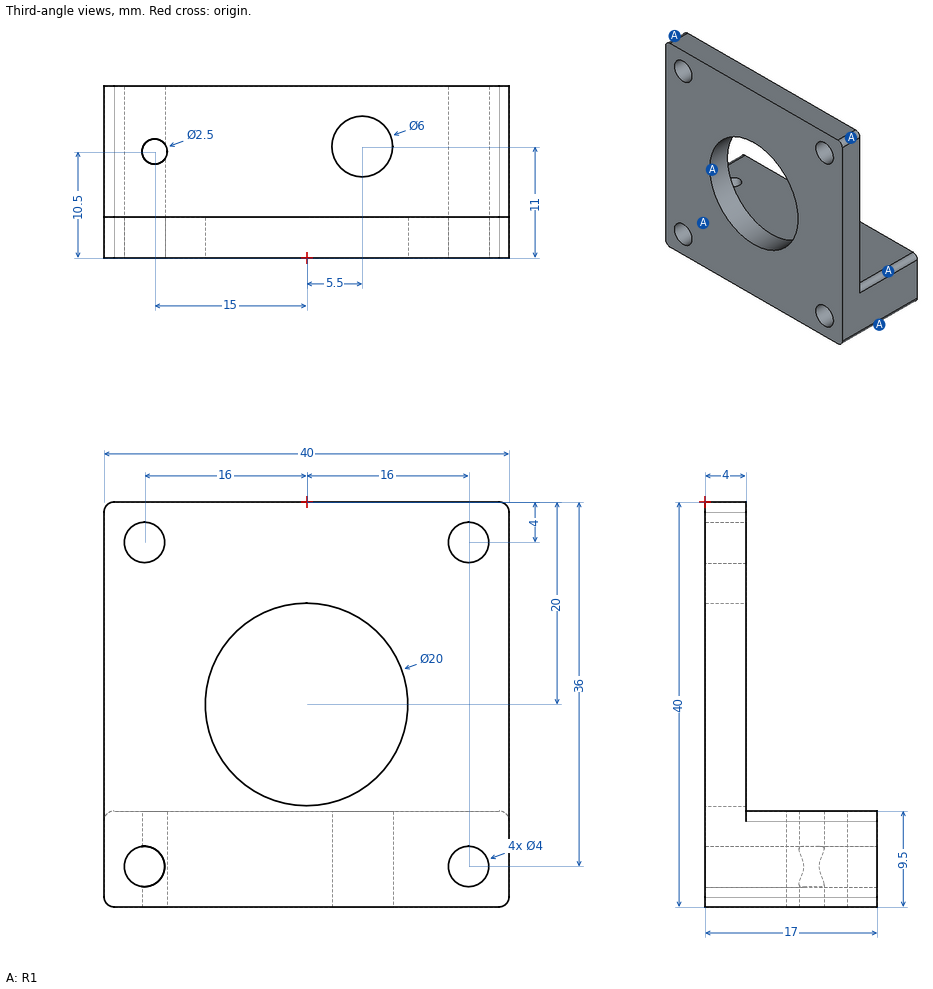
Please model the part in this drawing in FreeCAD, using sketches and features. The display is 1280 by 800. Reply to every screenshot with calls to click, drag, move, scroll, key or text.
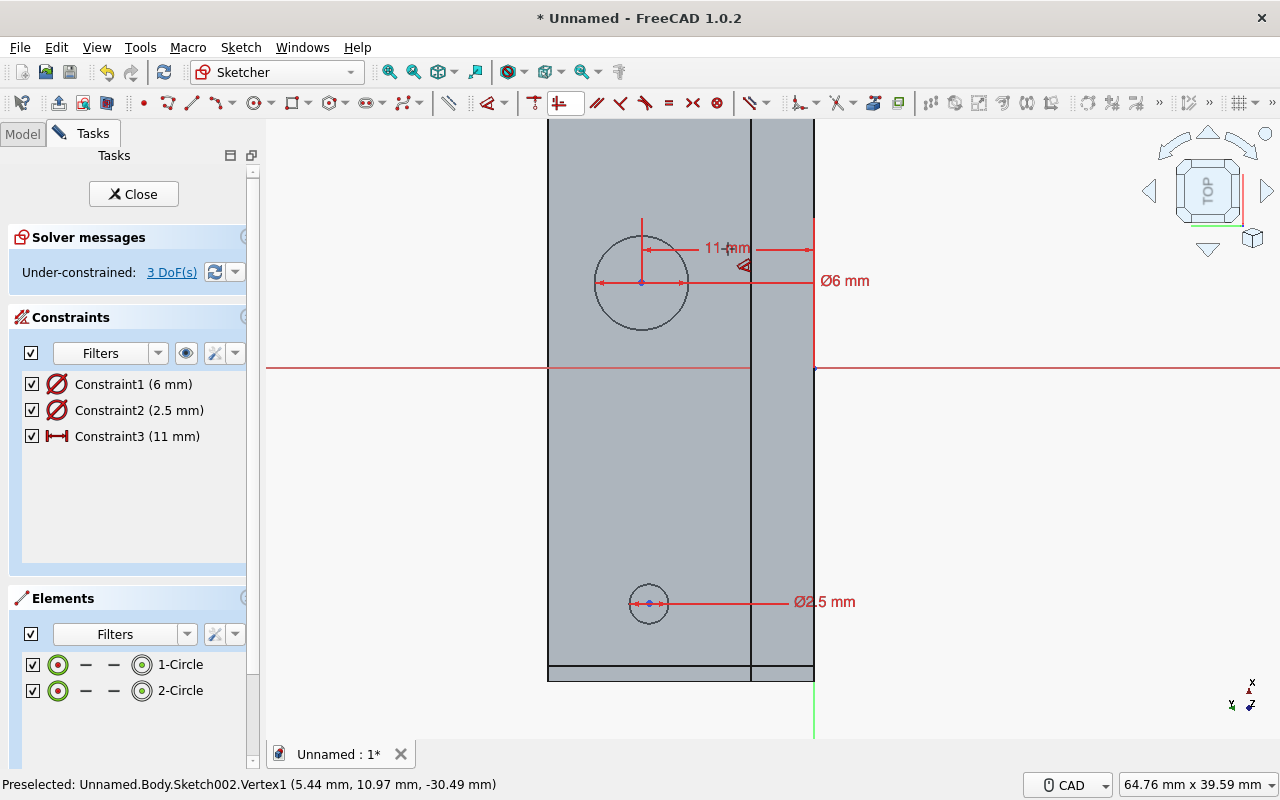
click(649, 604)
click(848, 486)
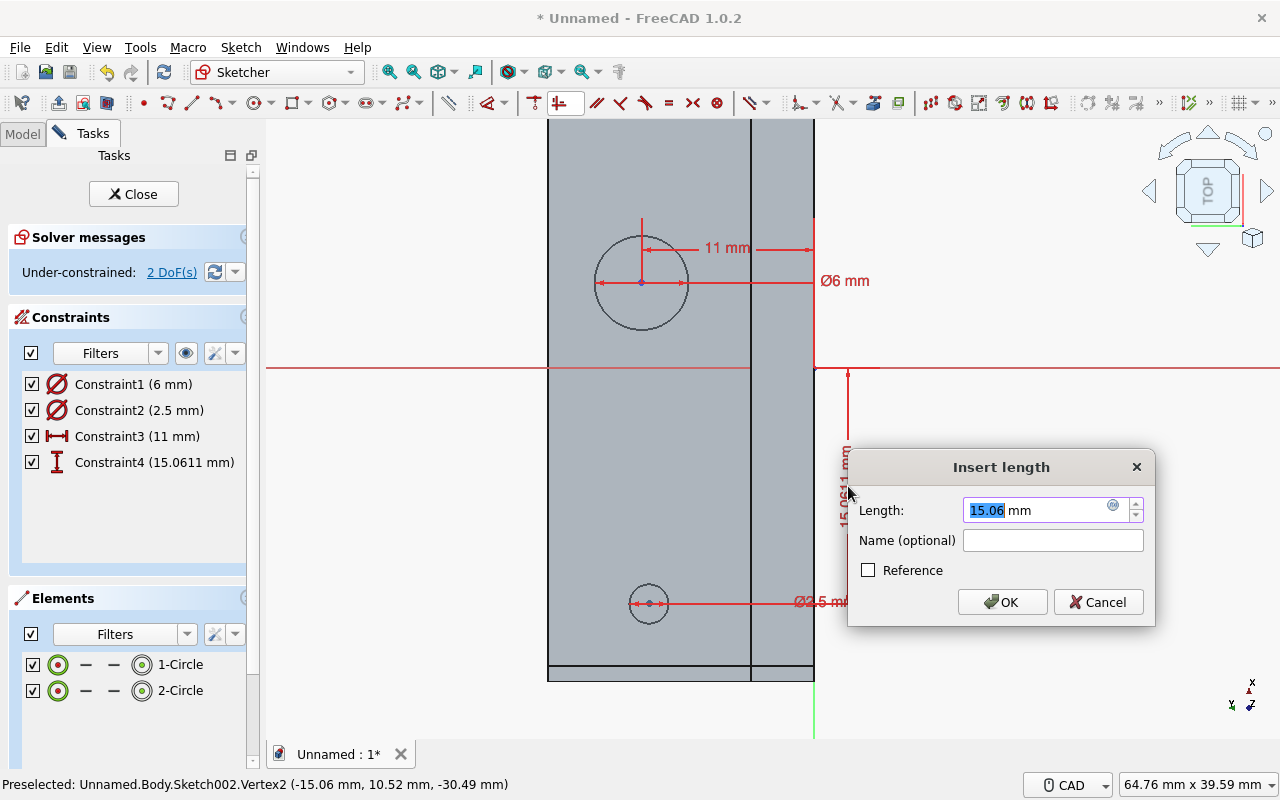
text(15)
key(Return)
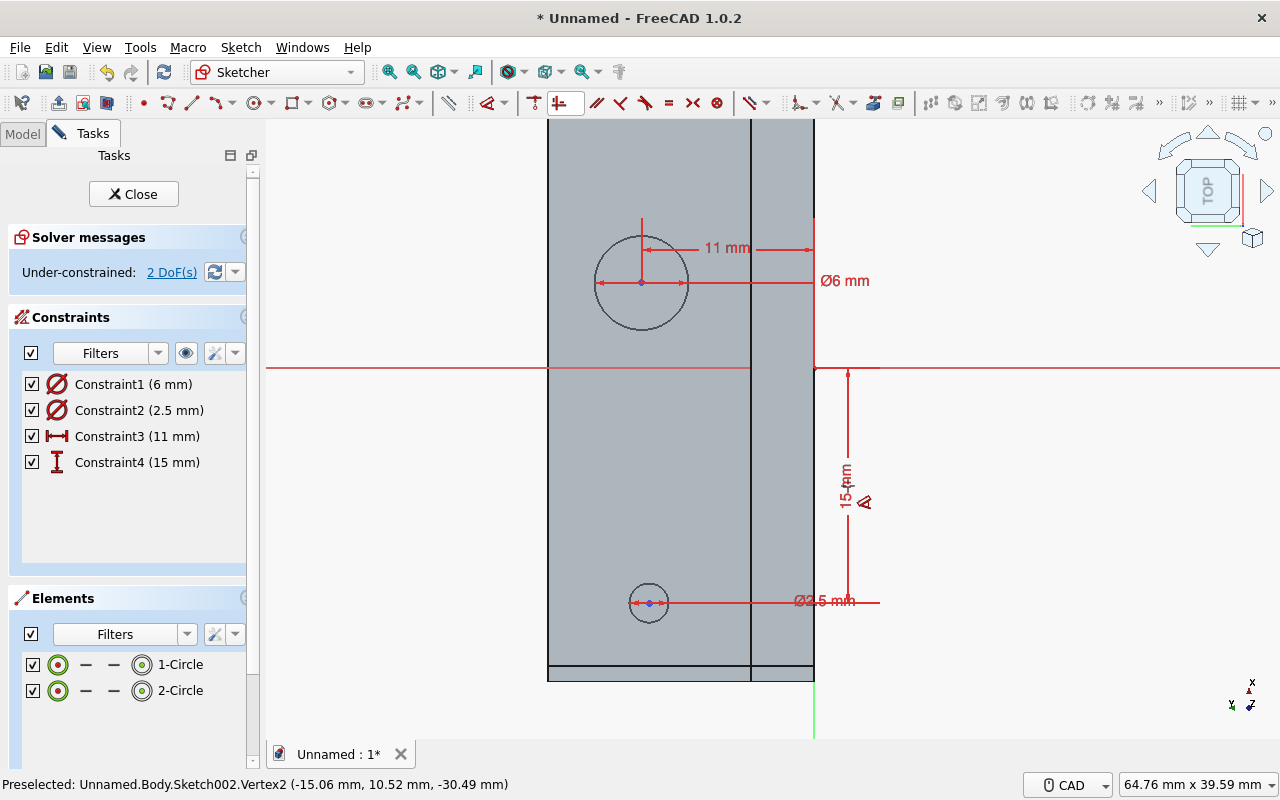
click(642, 283)
click(848, 326)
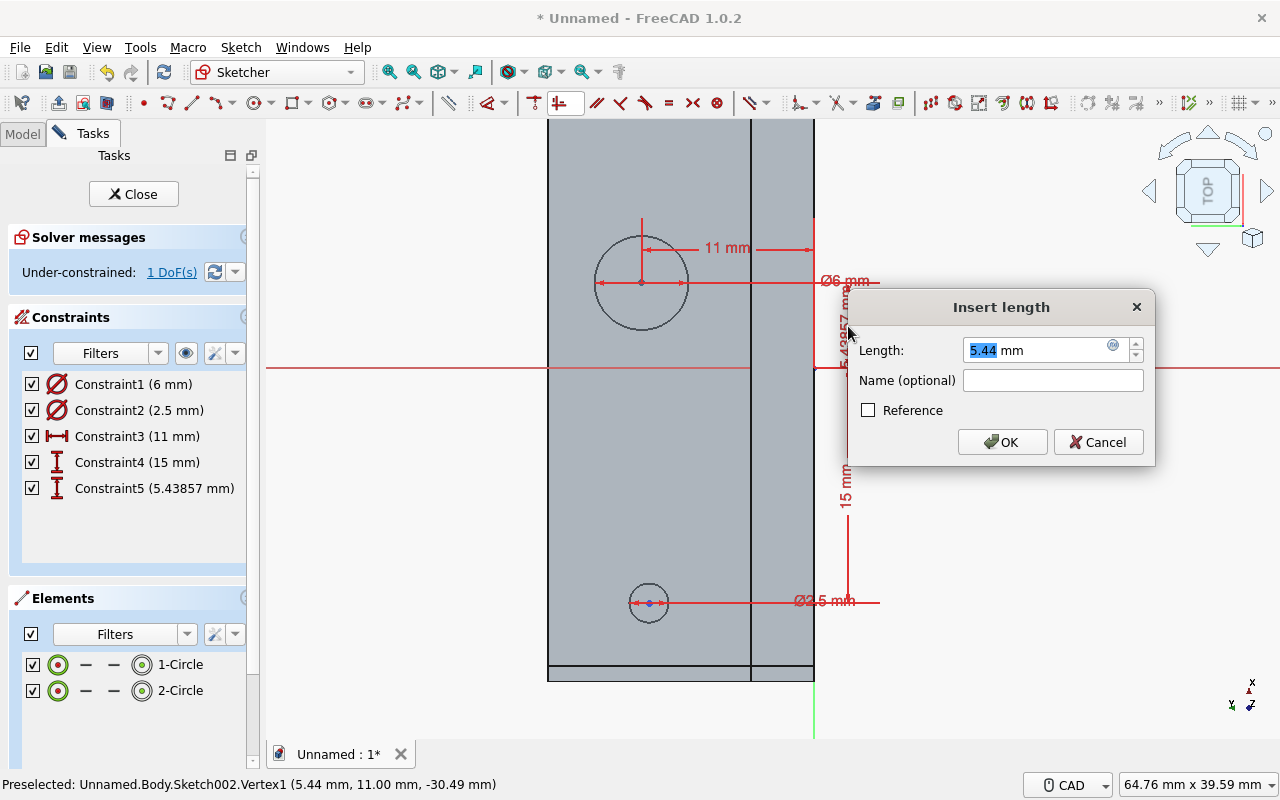
text(5.5)
key(Return)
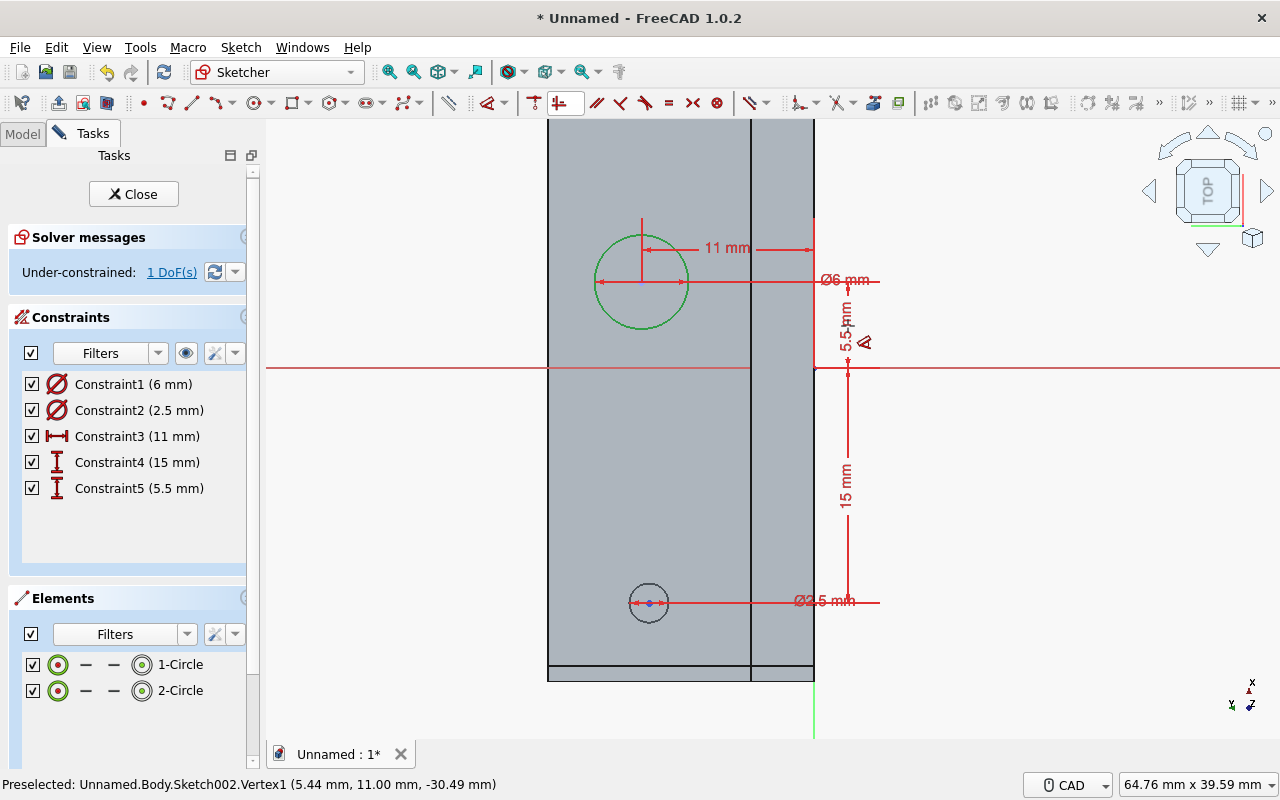
click(649, 603)
click(731, 637)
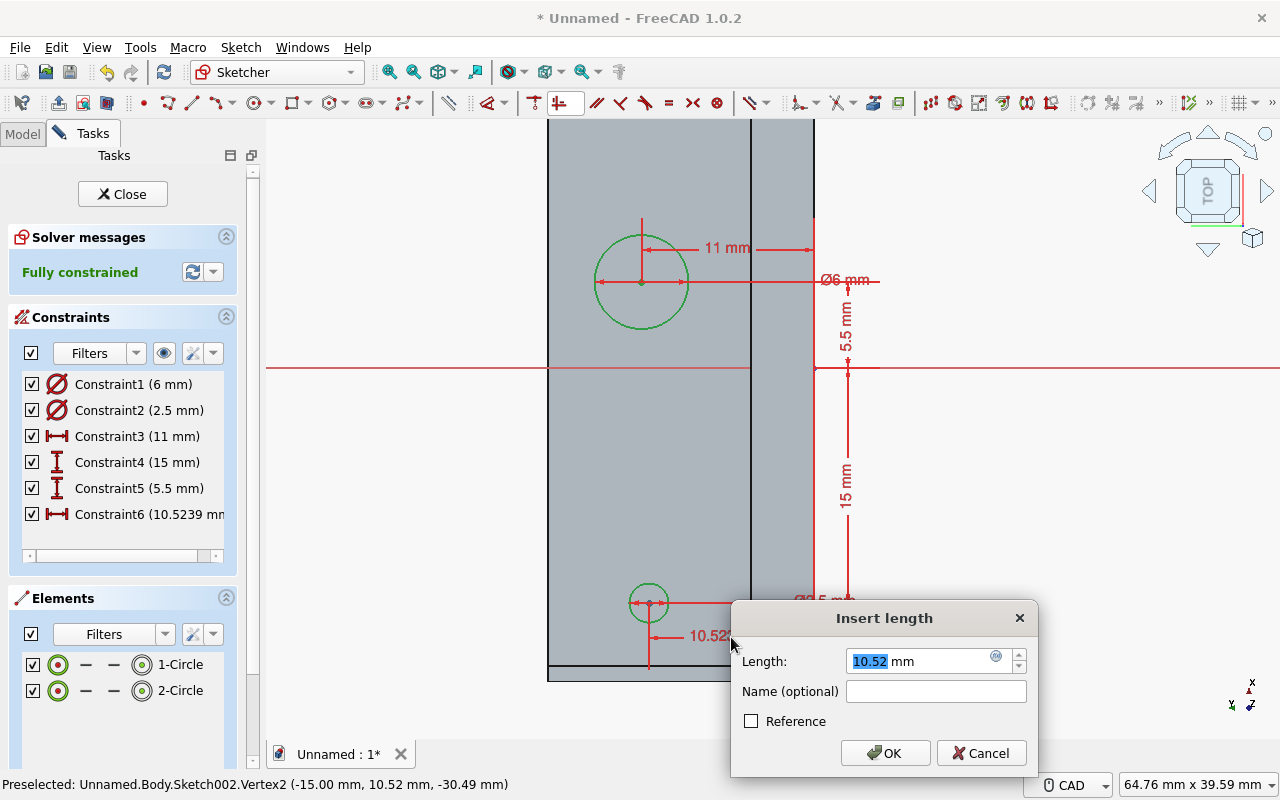
text(10.5)
key(Return)
key(Escape)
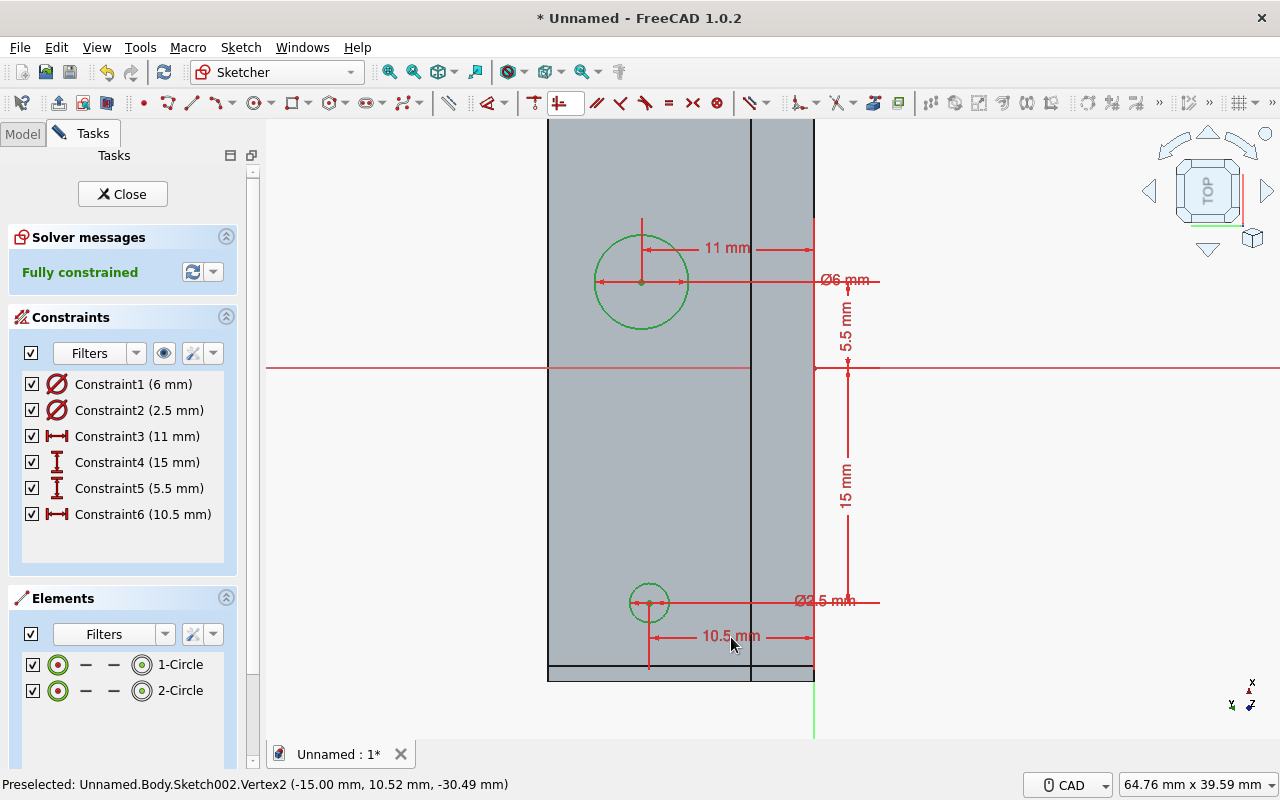
click(123, 194)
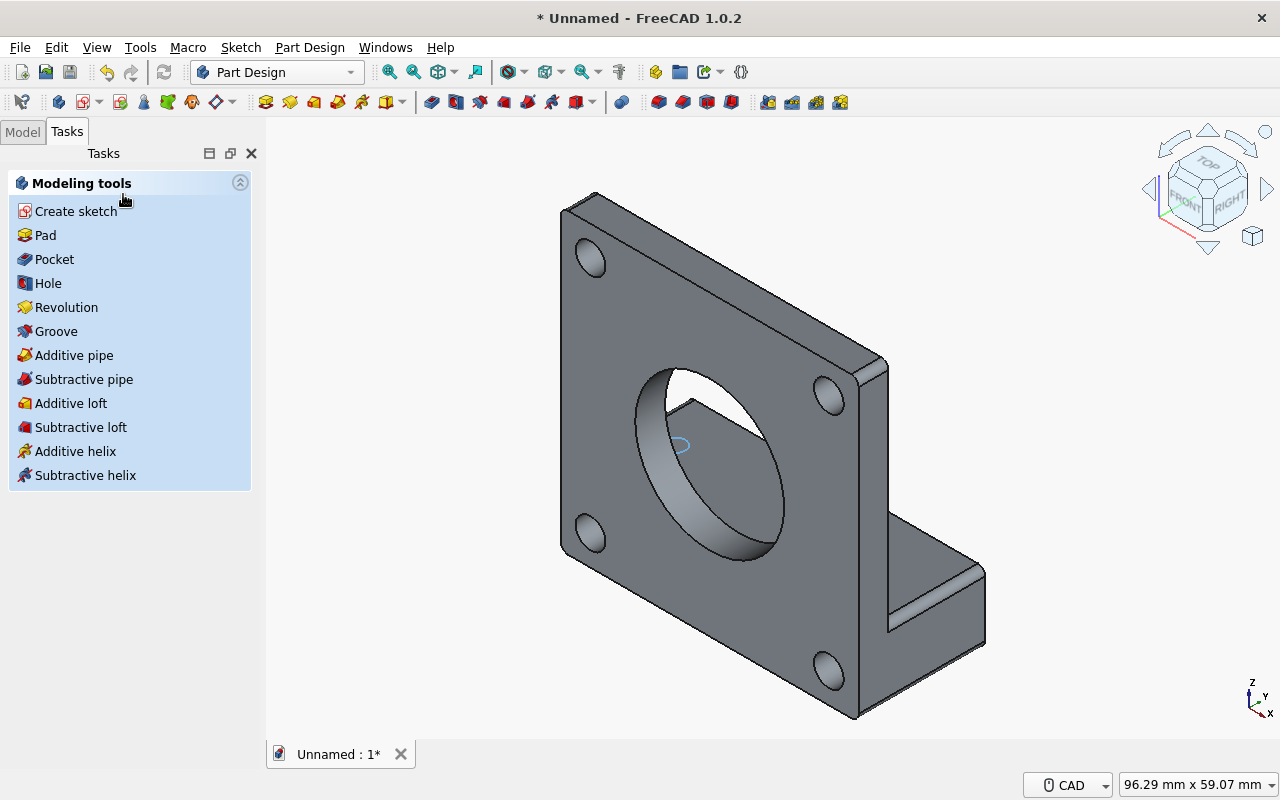
click(432, 102)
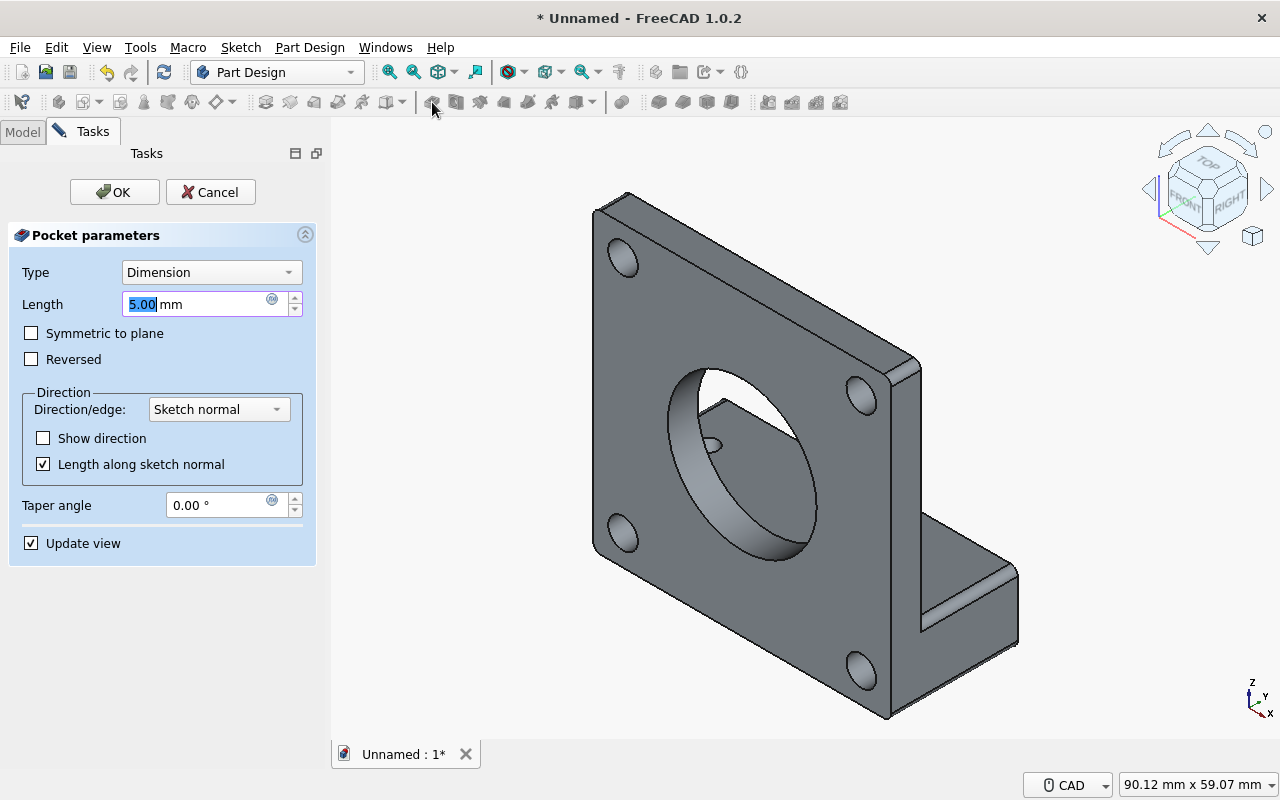
click(212, 272)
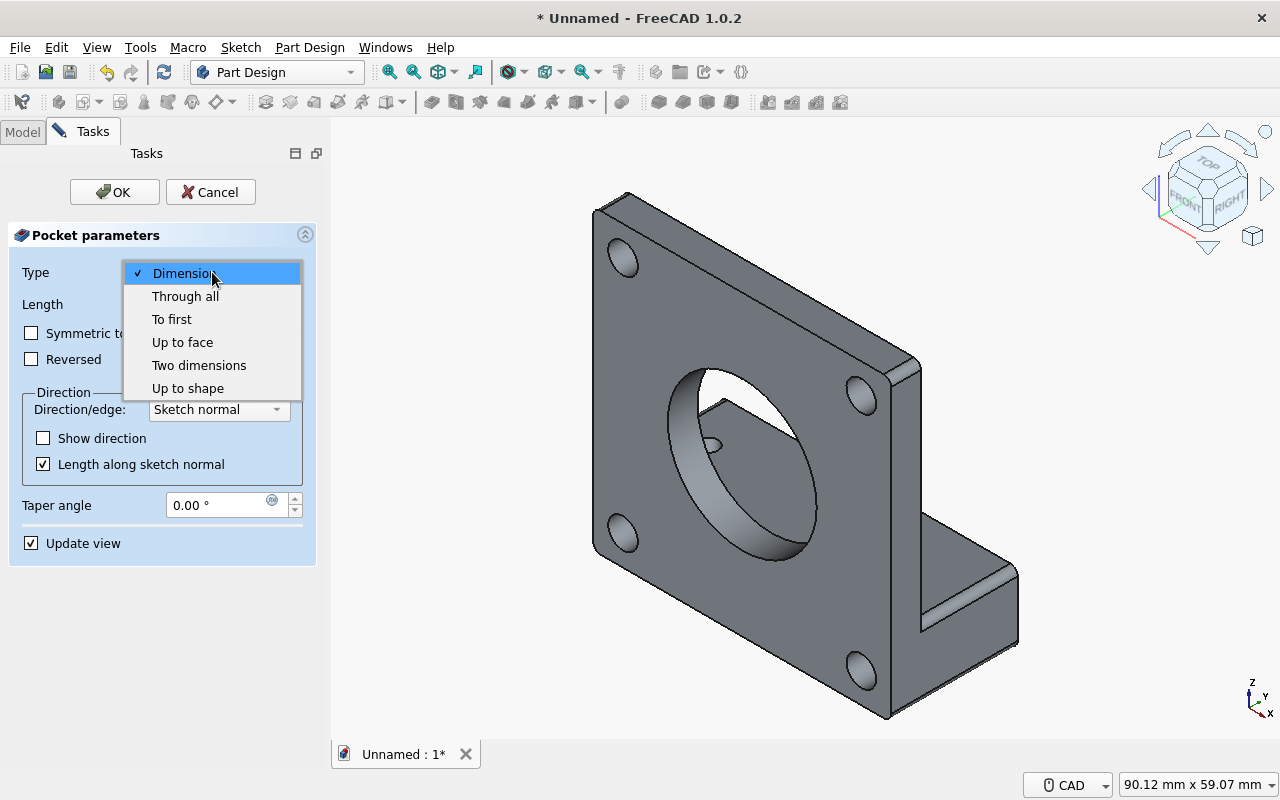
click(212, 296)